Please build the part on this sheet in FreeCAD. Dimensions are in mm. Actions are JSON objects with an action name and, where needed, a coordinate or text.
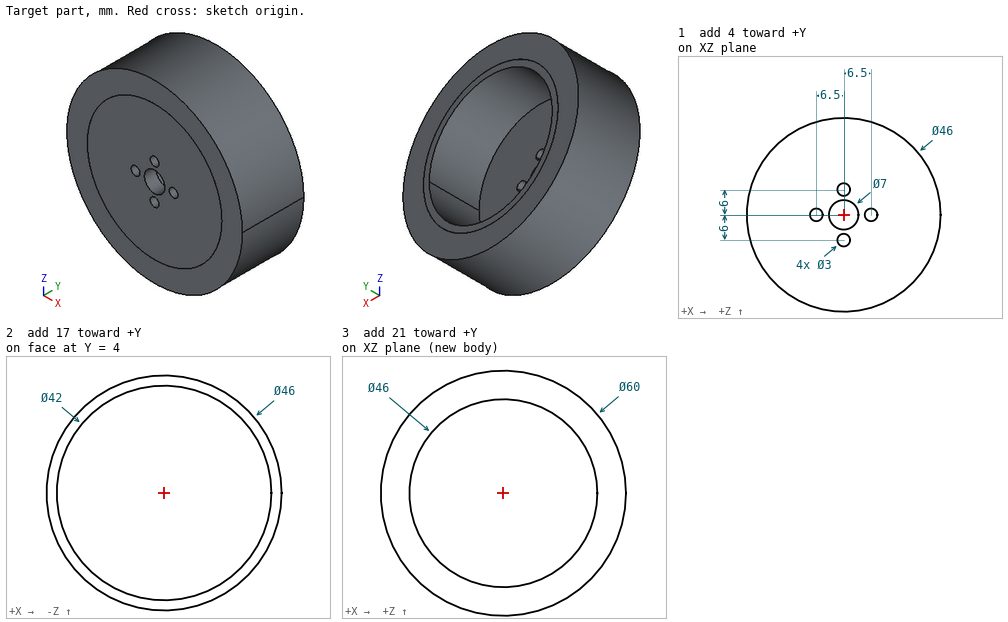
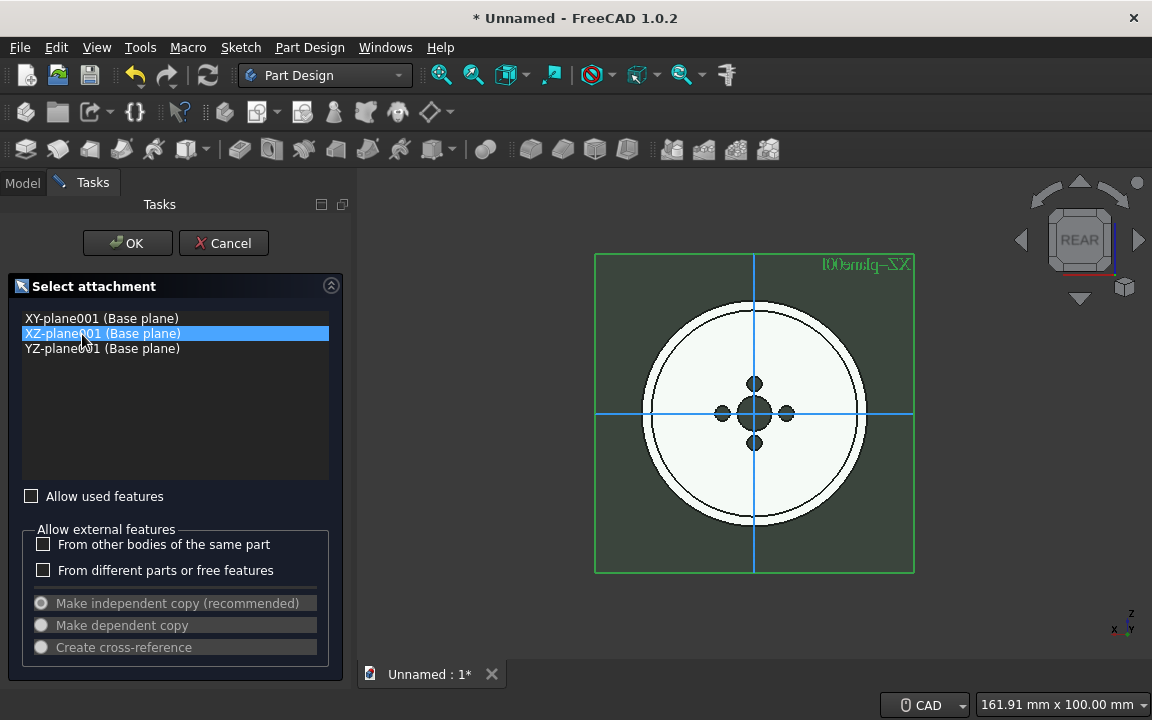
{"action": "left_click", "coordinate": [128, 243]}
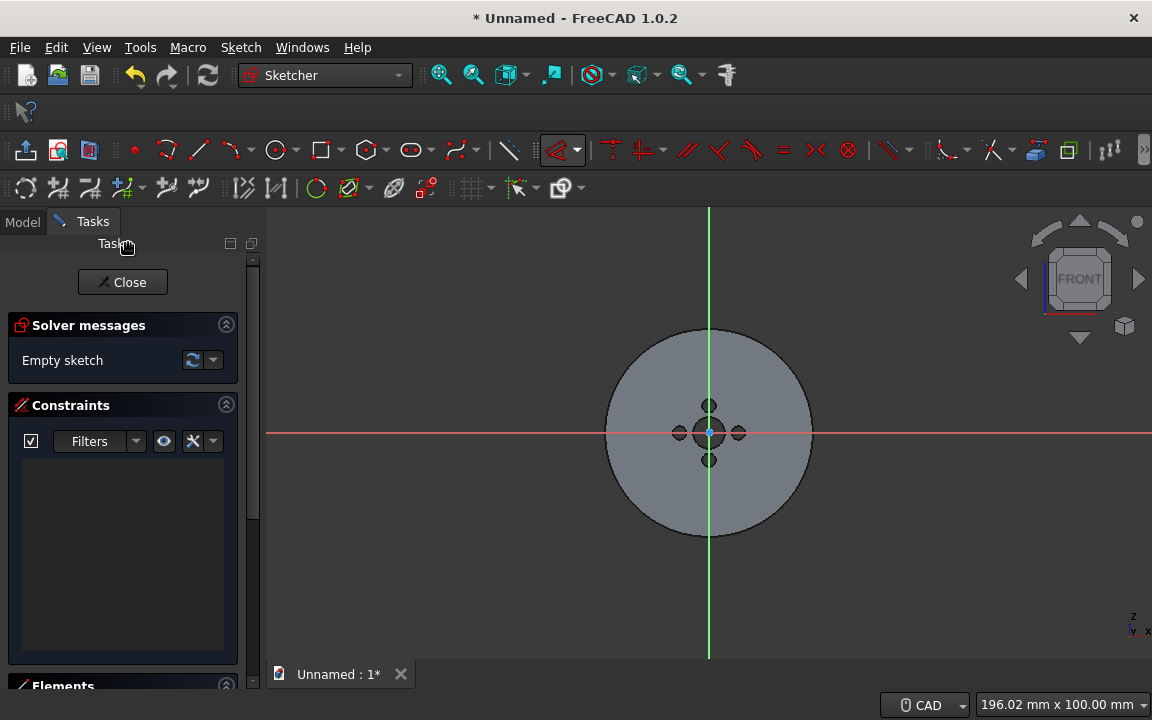
{"action": "left_click", "coordinate": [276, 150]}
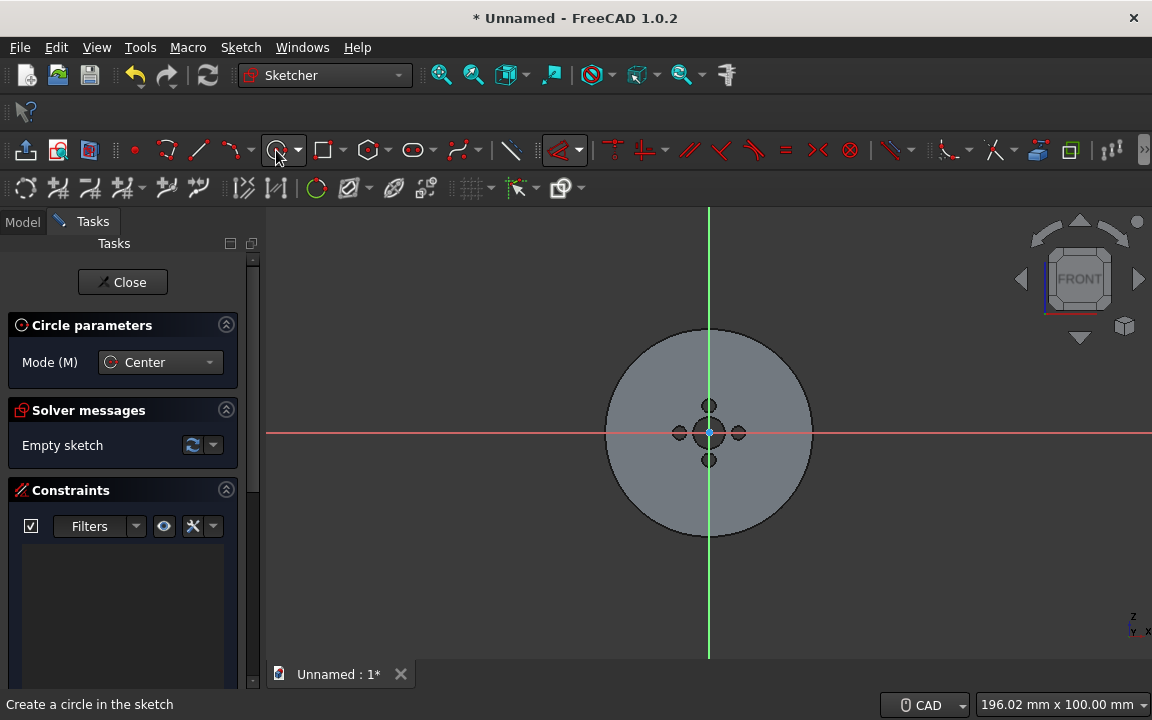
{"action": "left_click", "coordinate": [709, 433]}
{"action": "left_click", "coordinate": [805, 337]}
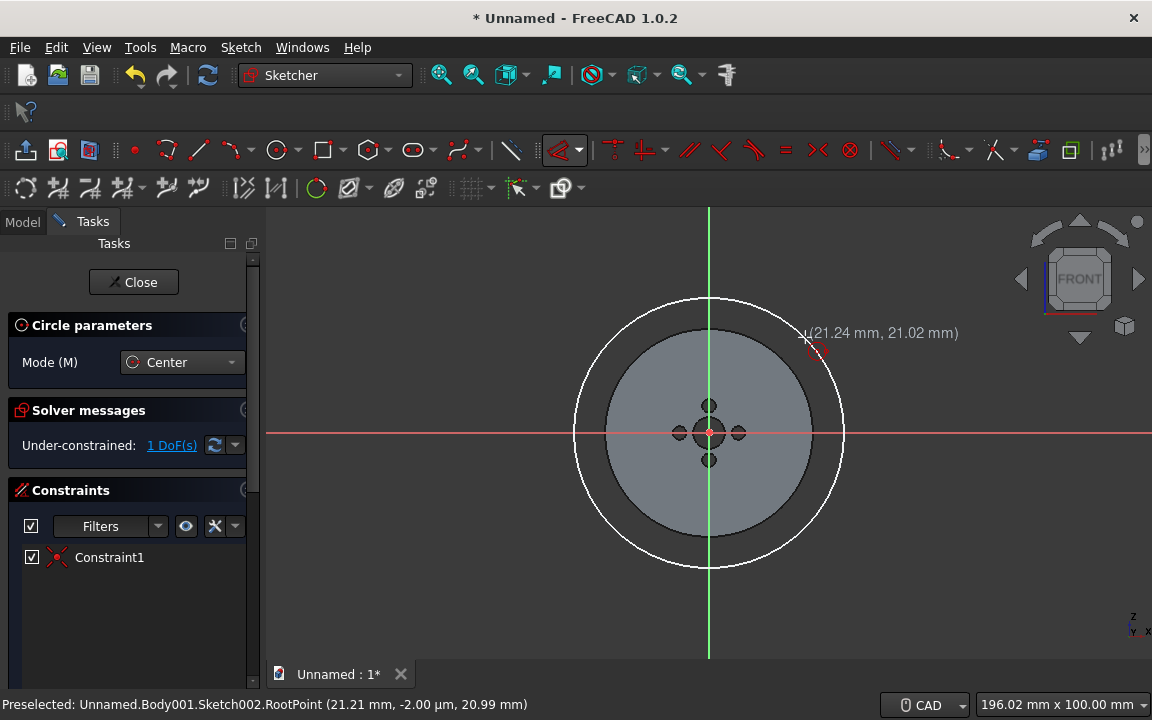
{"action": "left_click", "coordinate": [709, 433]}
{"action": "left_click", "coordinate": [783, 359]}
{"action": "key", "text": "Escape"}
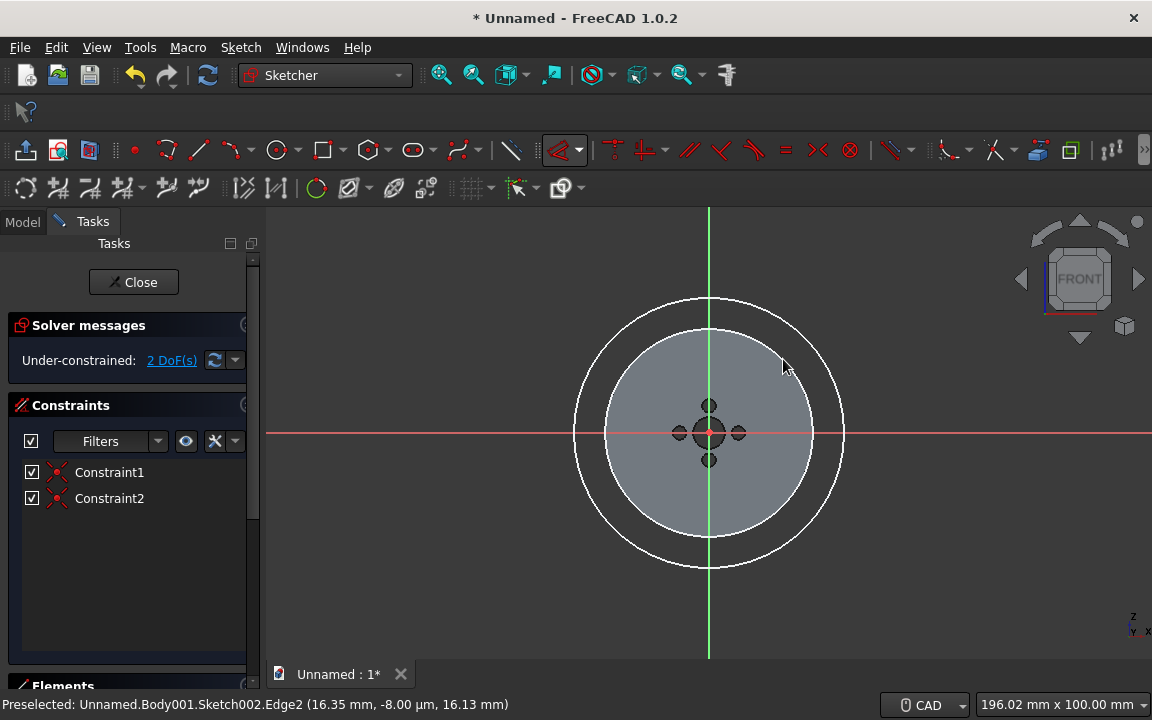
{"action": "left_click", "coordinate": [804, 337]}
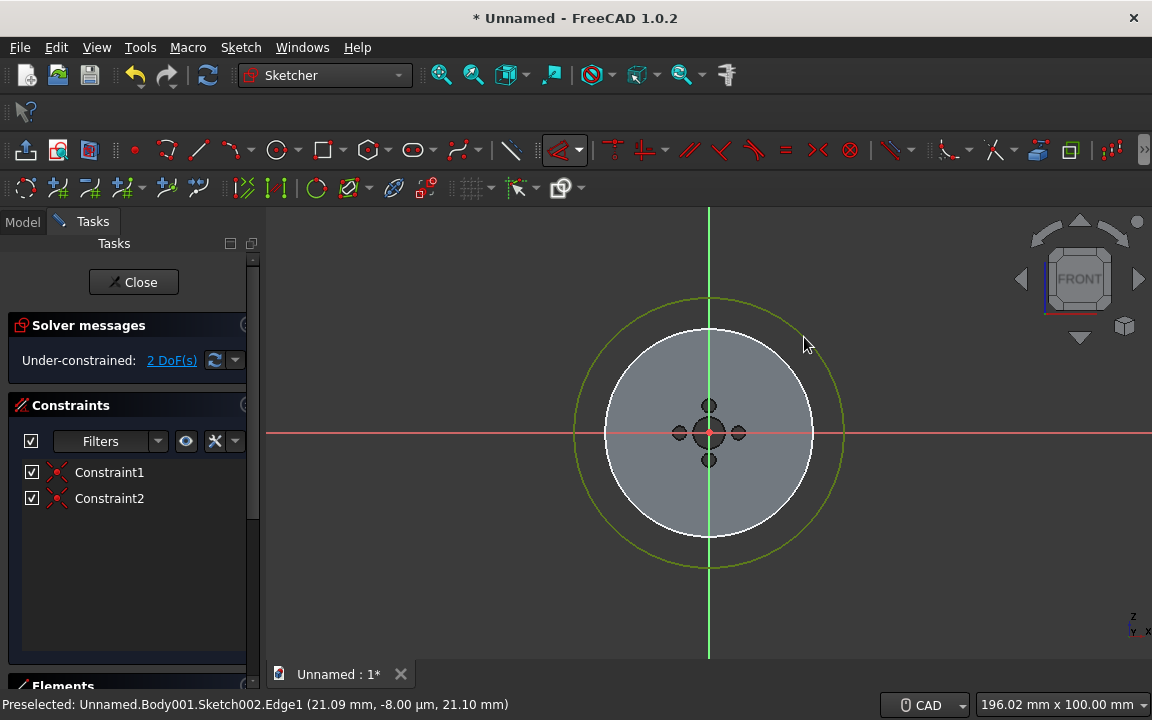
{"action": "left_click", "coordinate": [582, 150]}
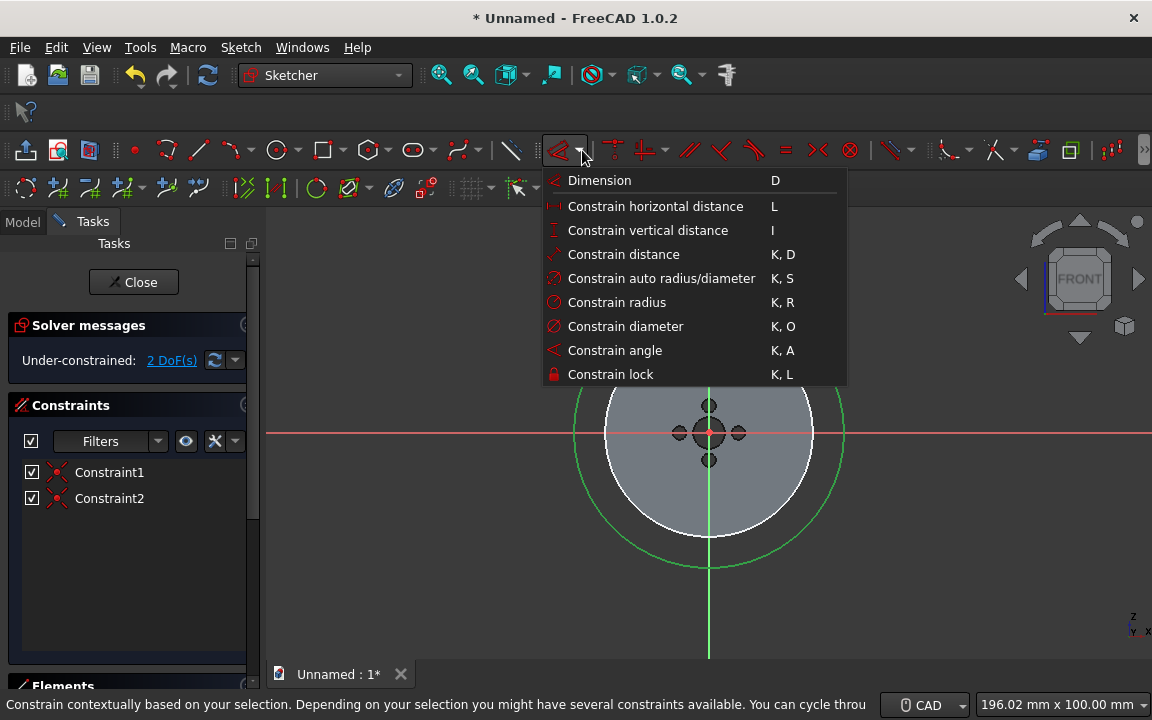
{"action": "left_click", "coordinate": [695, 326]}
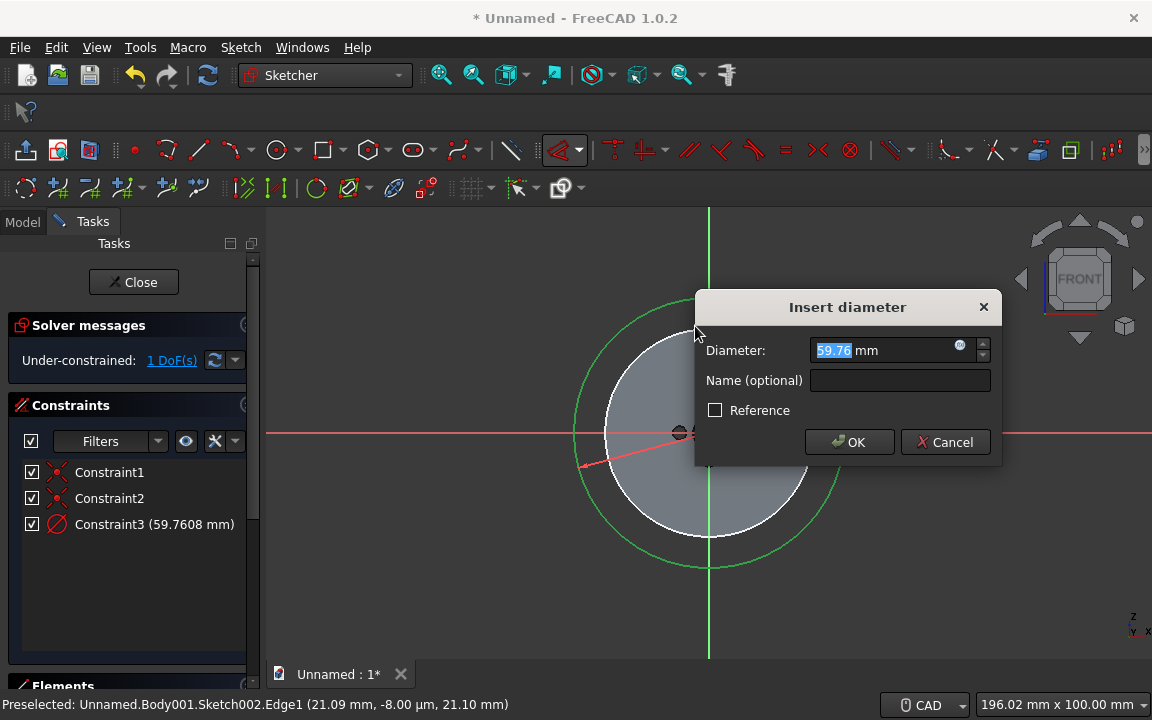
{"action": "type", "text": "60"}
{"action": "key", "text": "Return"}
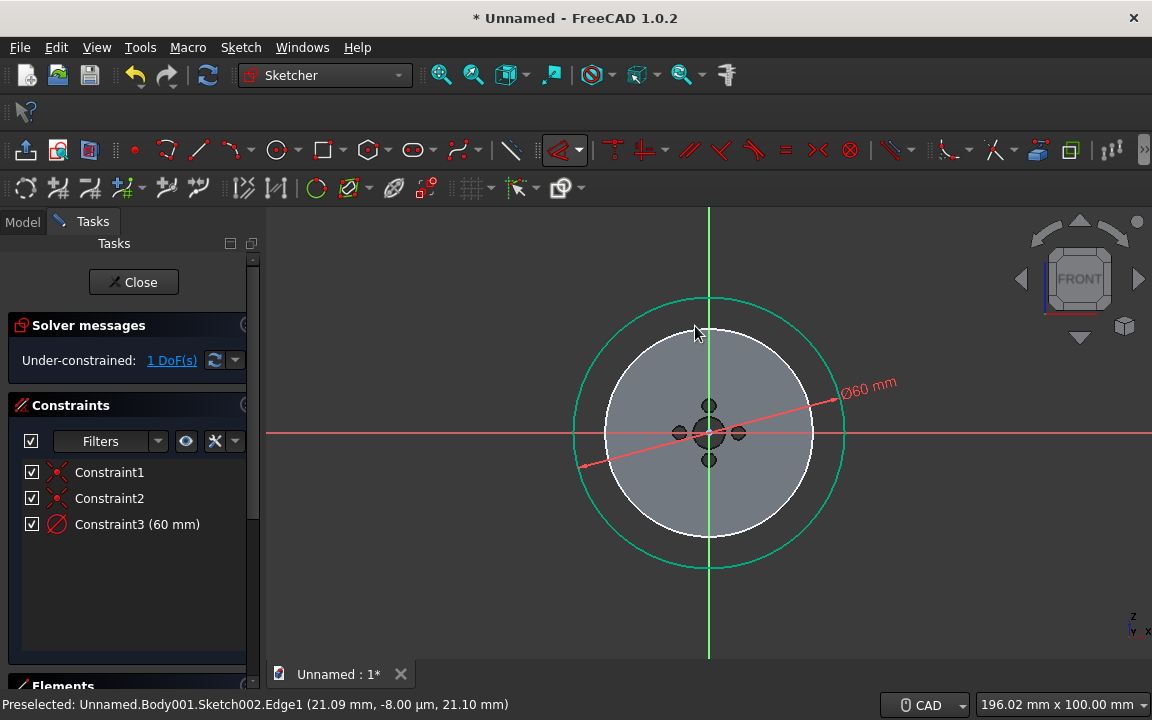
{"action": "left_click", "coordinate": [782, 359]}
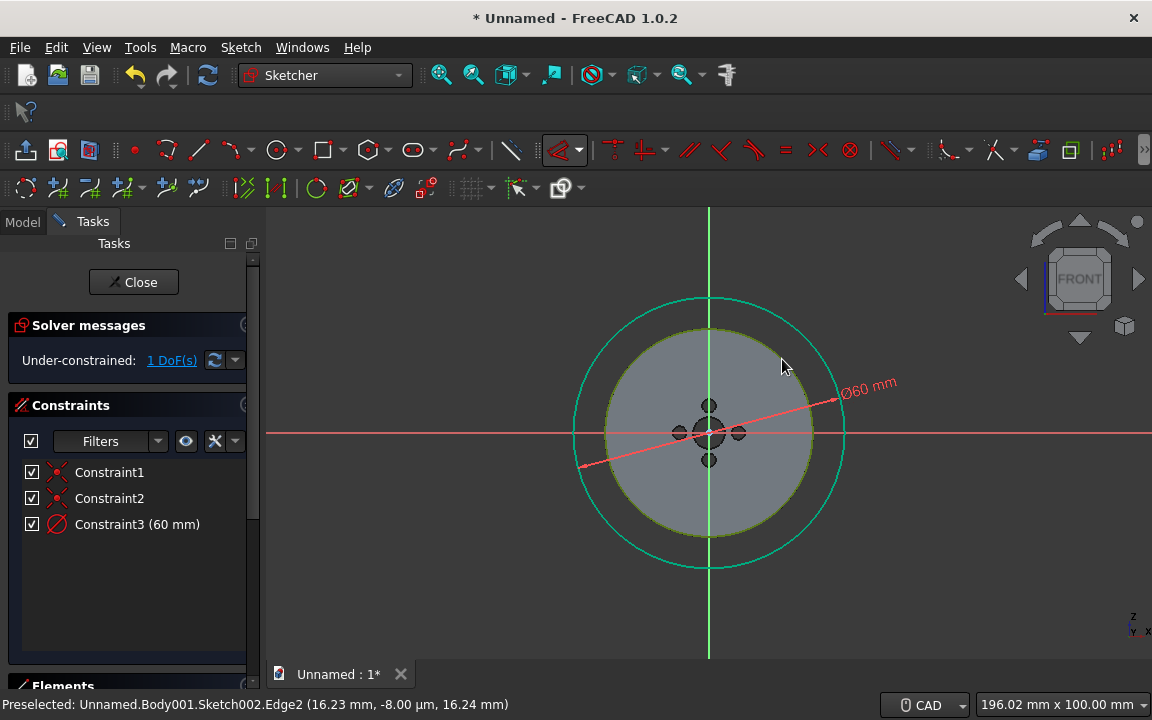
{"action": "key", "text": "k o"}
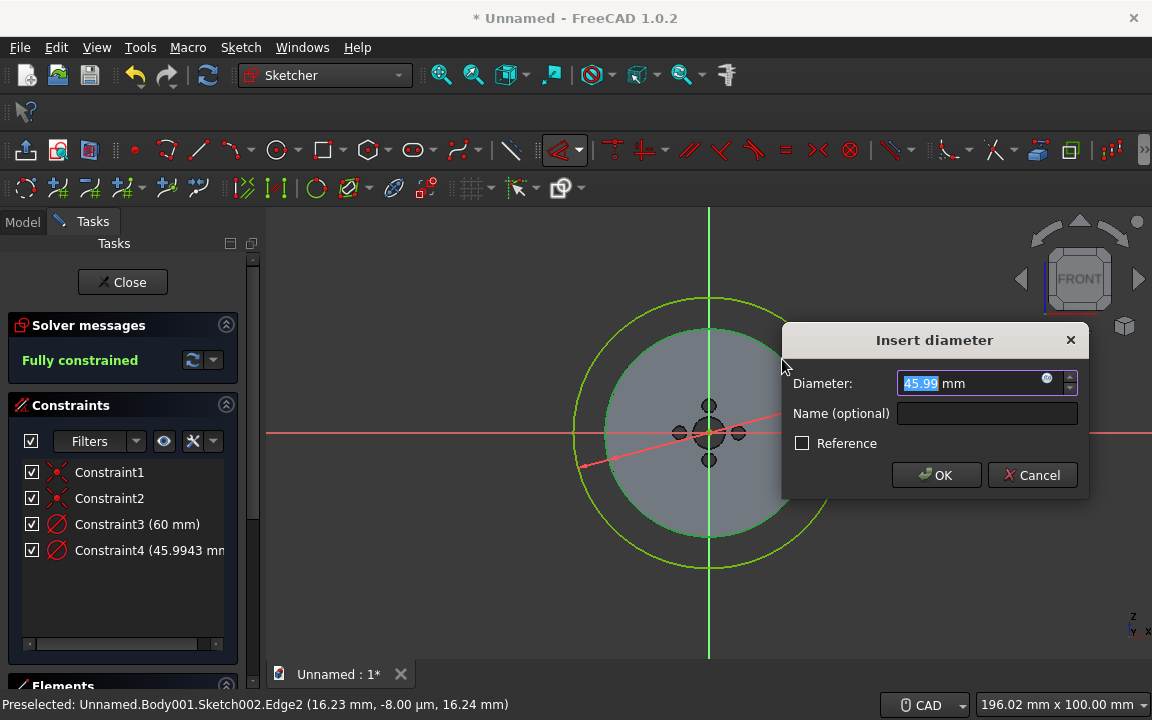
{"action": "type", "text": "46"}
{"action": "key", "text": "Return"}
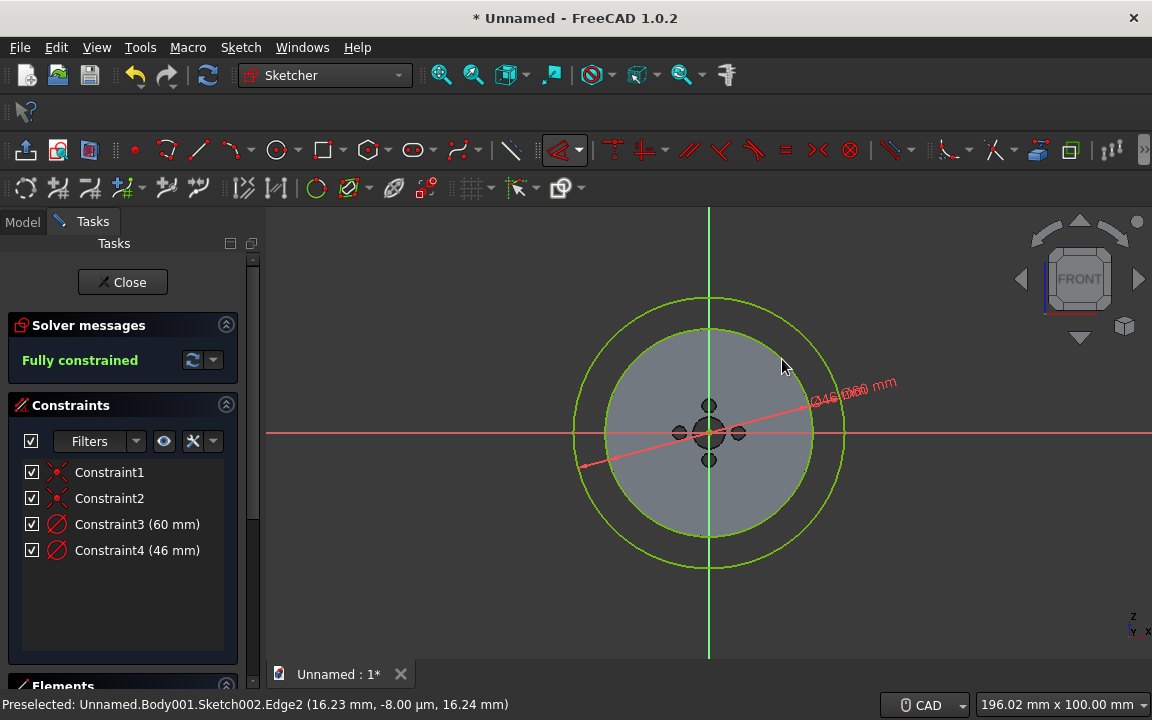
{"action": "left_click", "coordinate": [123, 282]}